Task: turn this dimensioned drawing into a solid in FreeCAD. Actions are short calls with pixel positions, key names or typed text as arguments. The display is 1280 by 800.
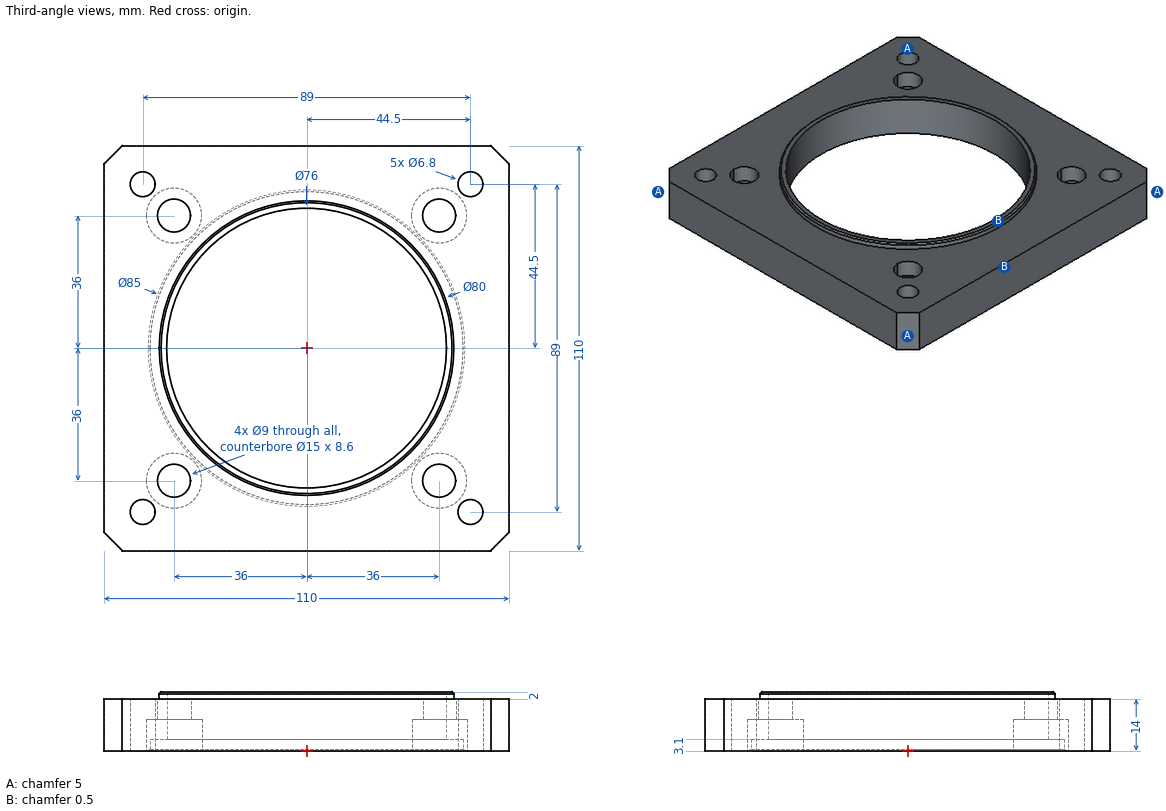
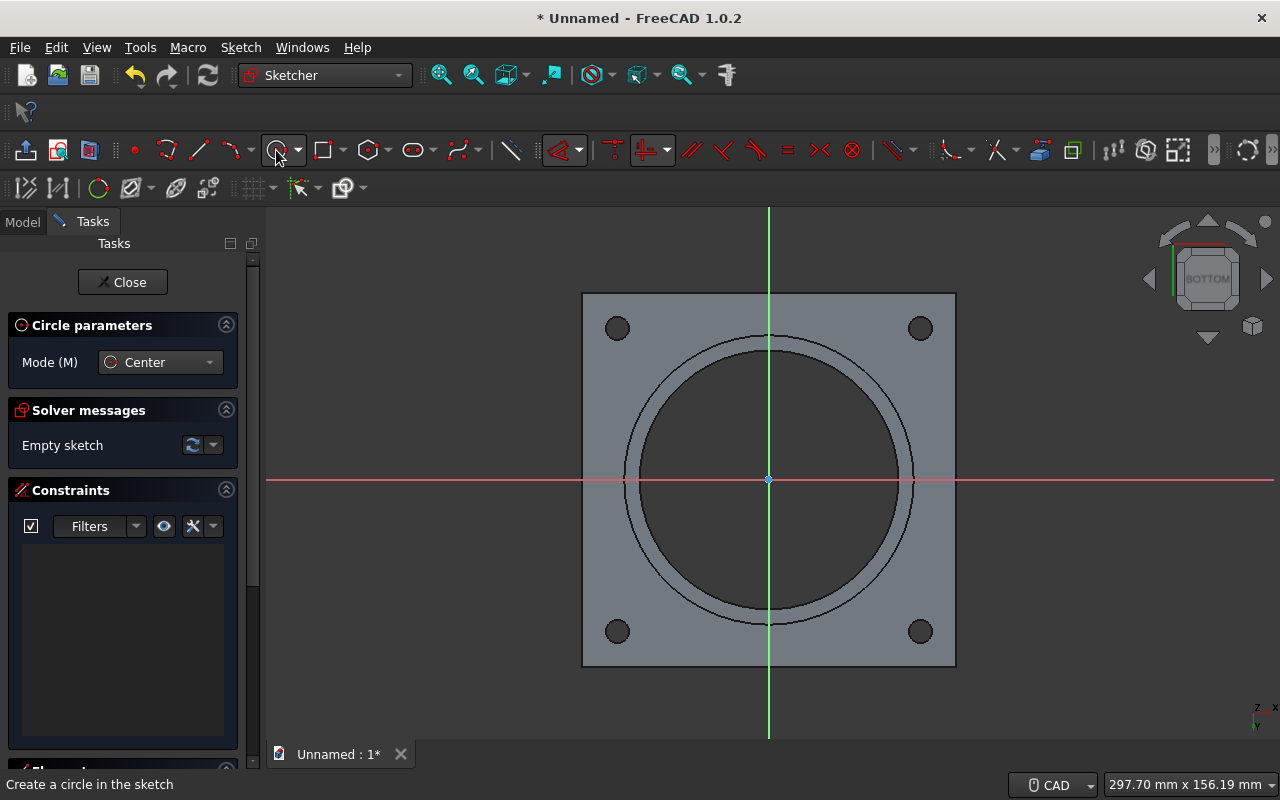
scroll(646, 357, up, 2)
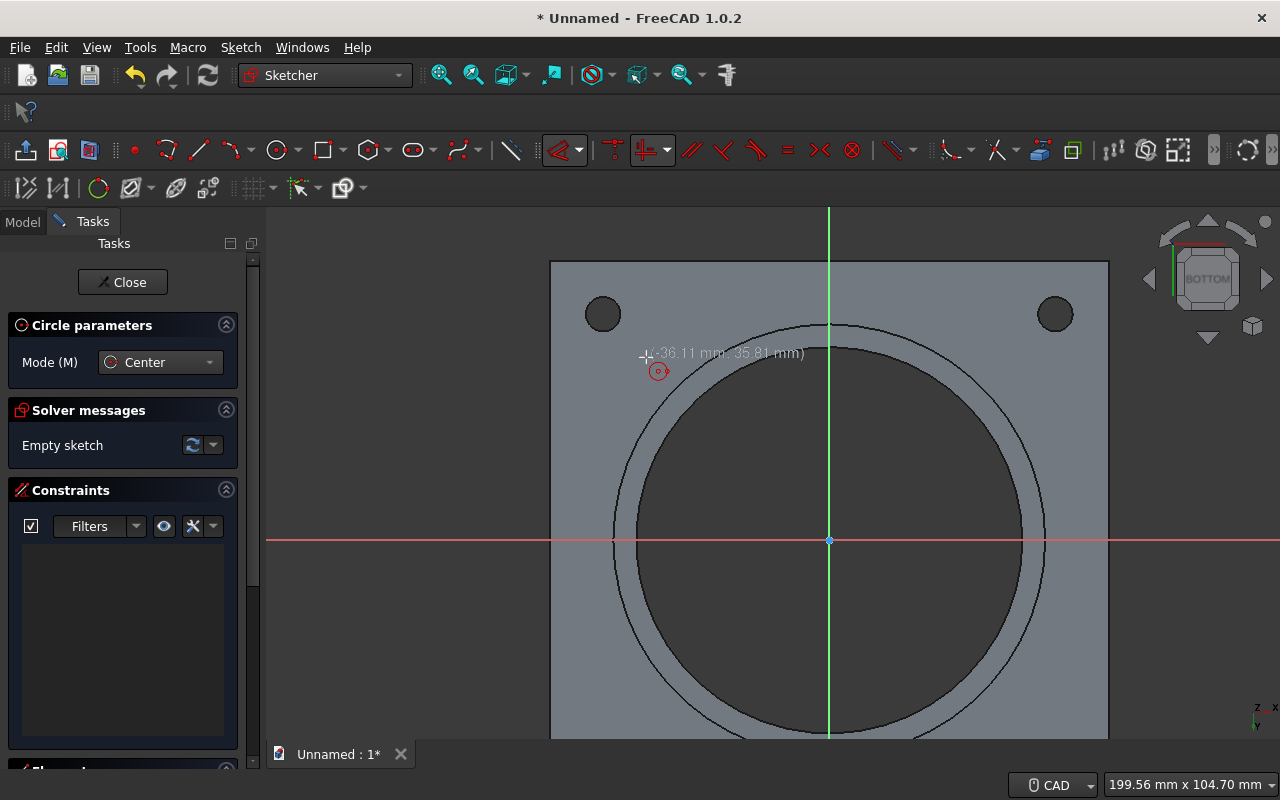
click(646, 357)
click(663, 341)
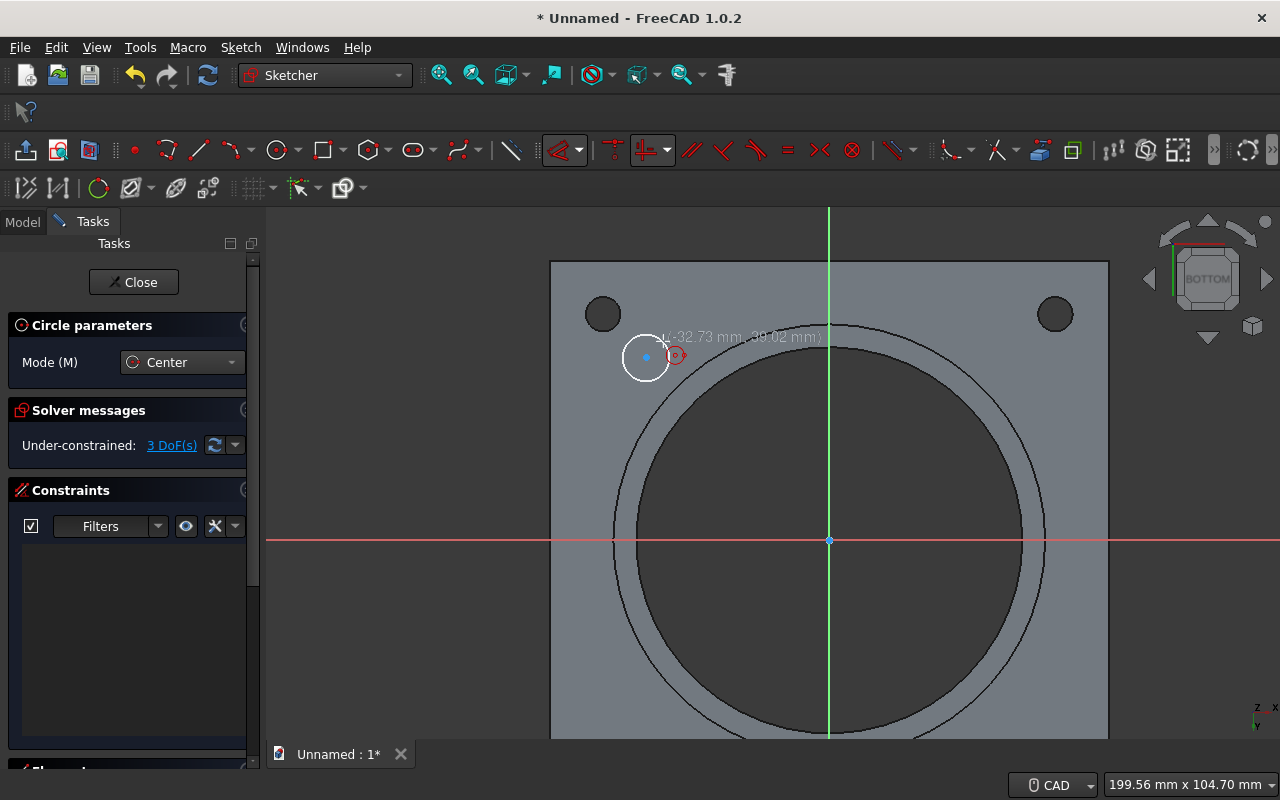
scroll(294, 235, down, 1)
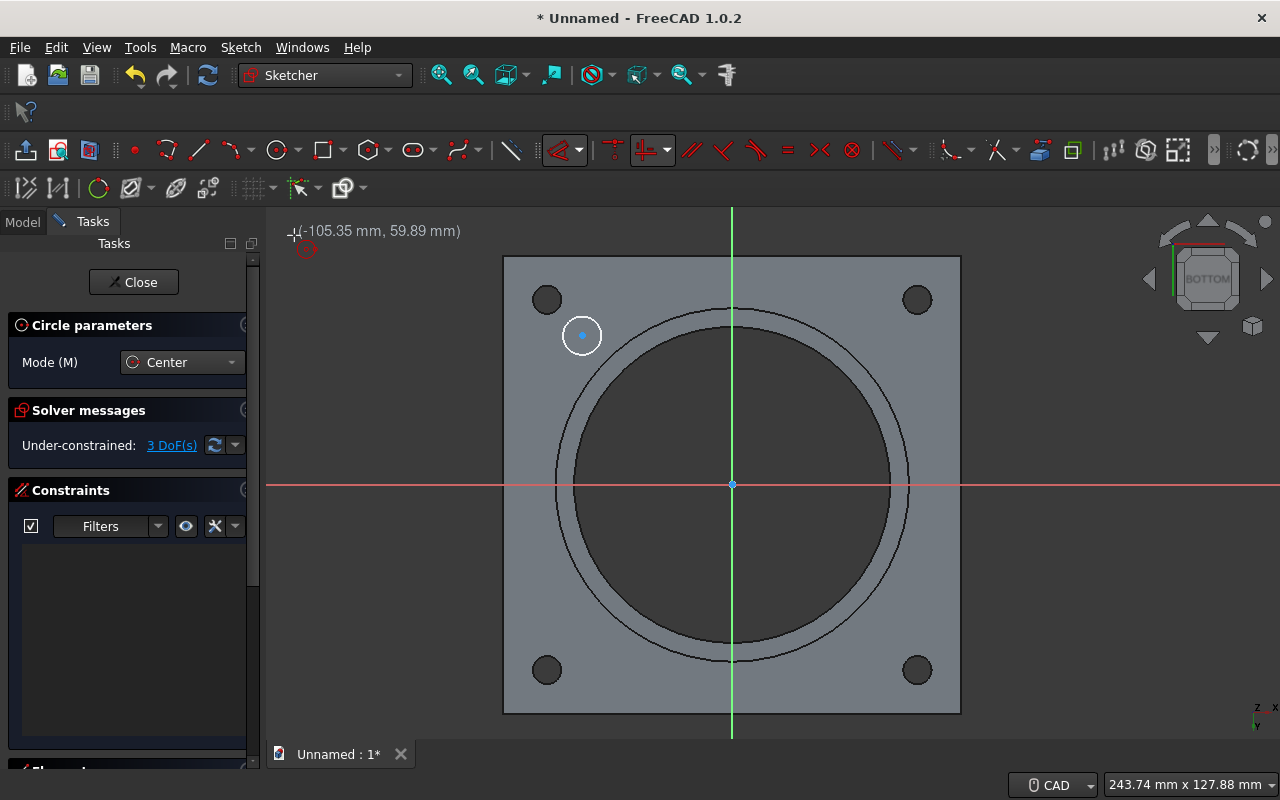
click(582, 635)
click(596, 621)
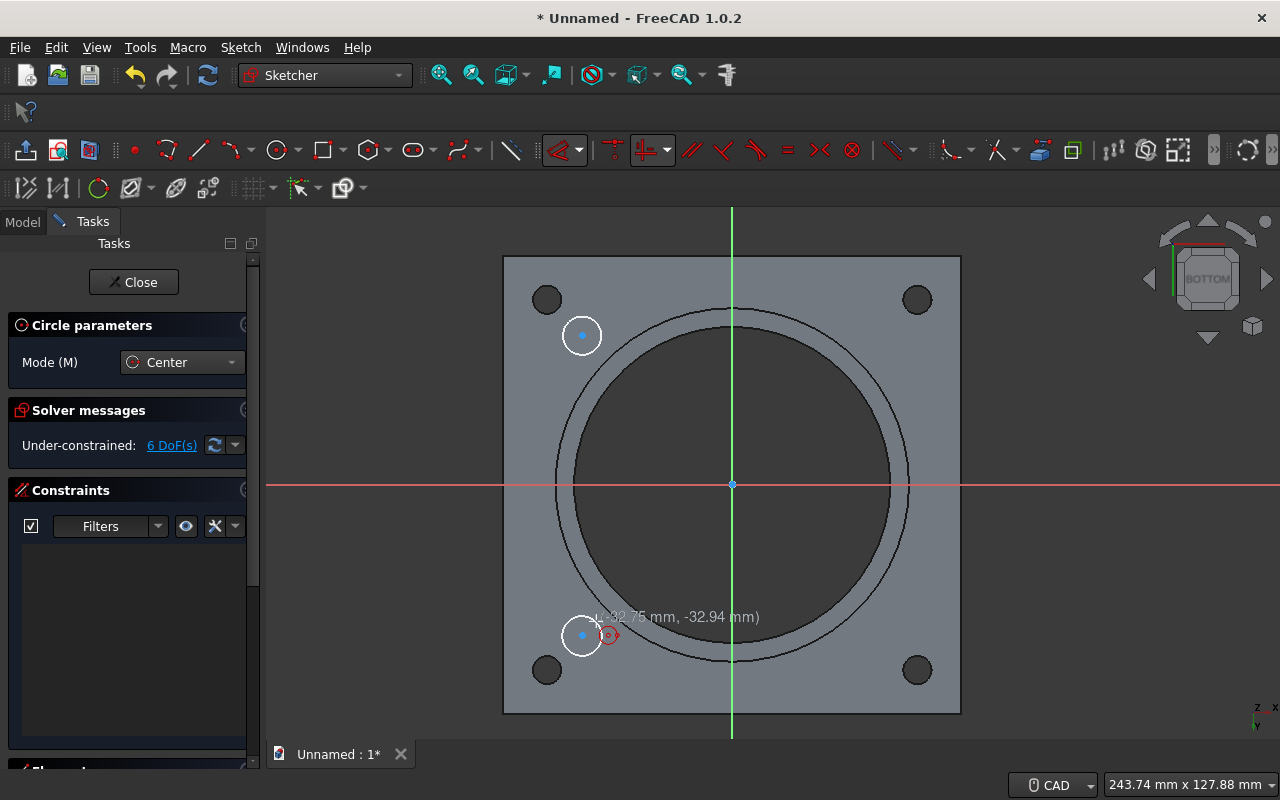
click(882, 335)
click(895, 322)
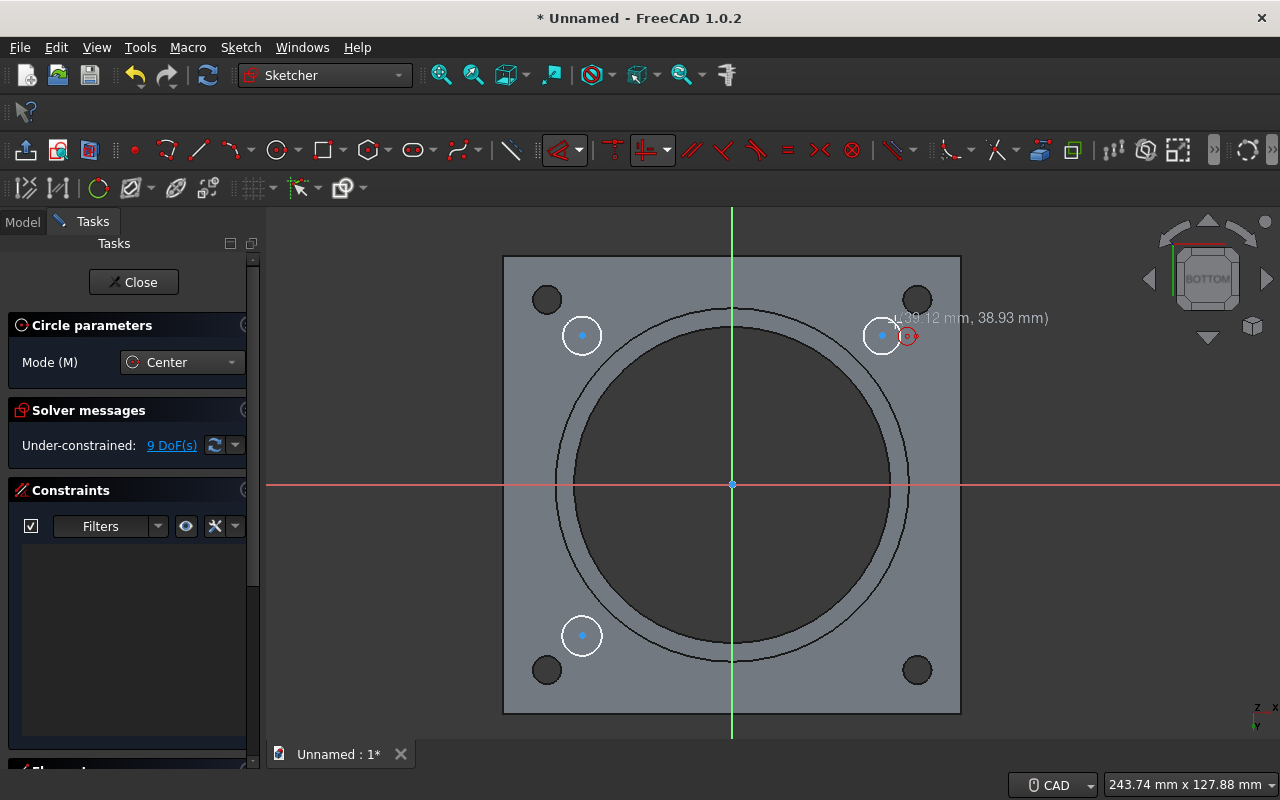
click(882, 635)
click(895, 621)
key(Escape)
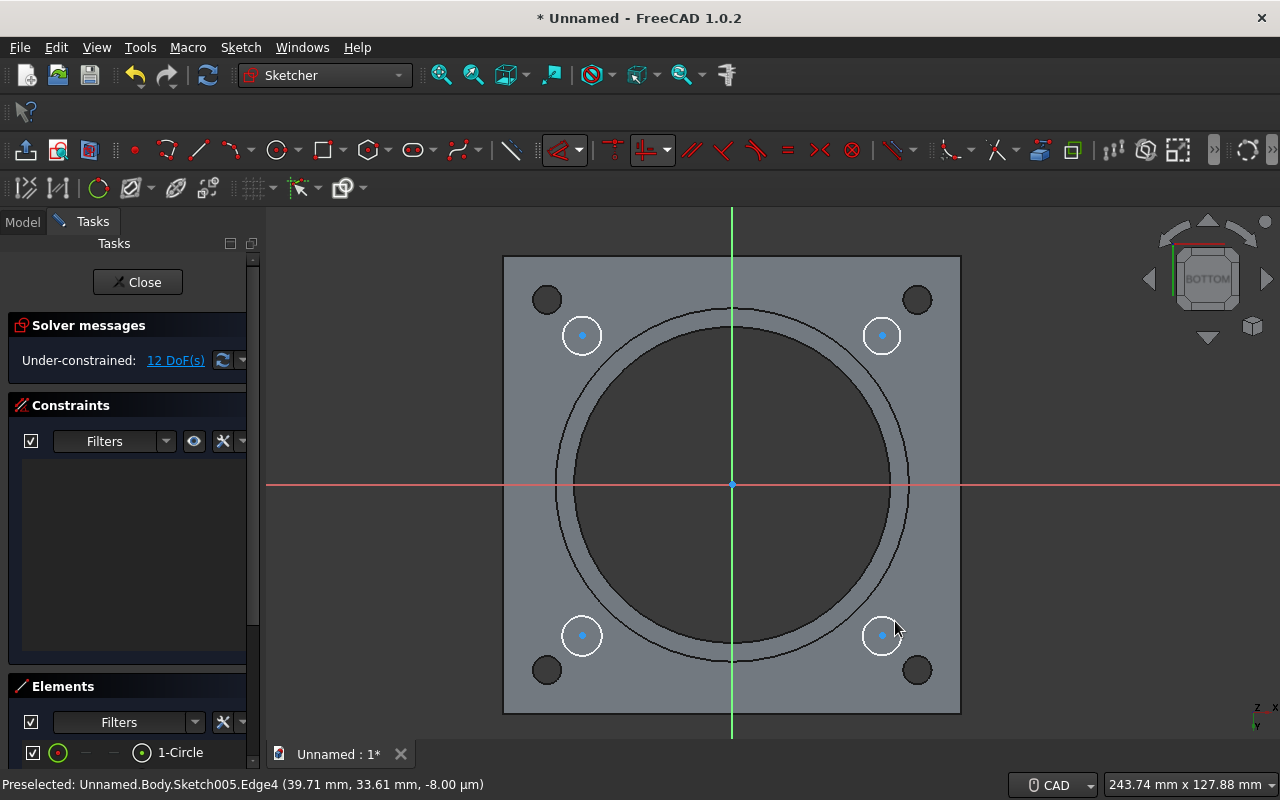
click(596, 322)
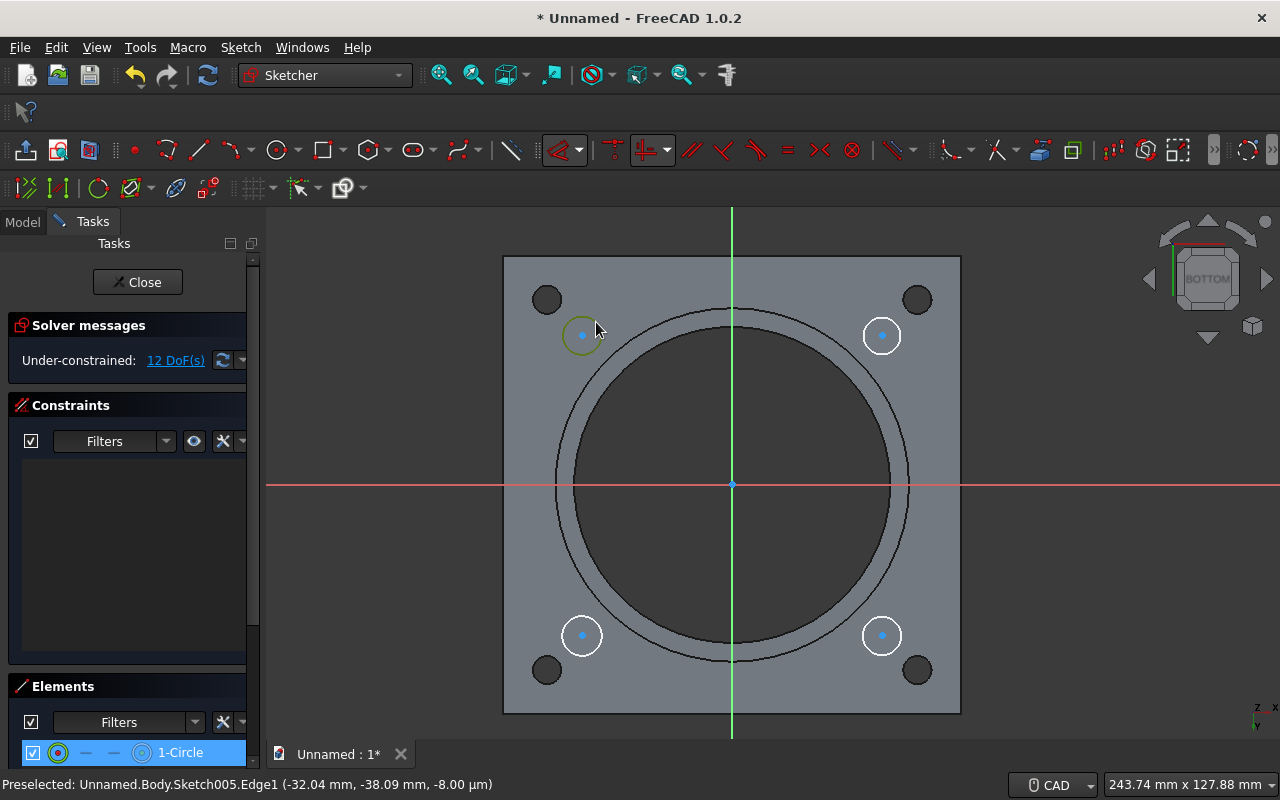
click(596, 622)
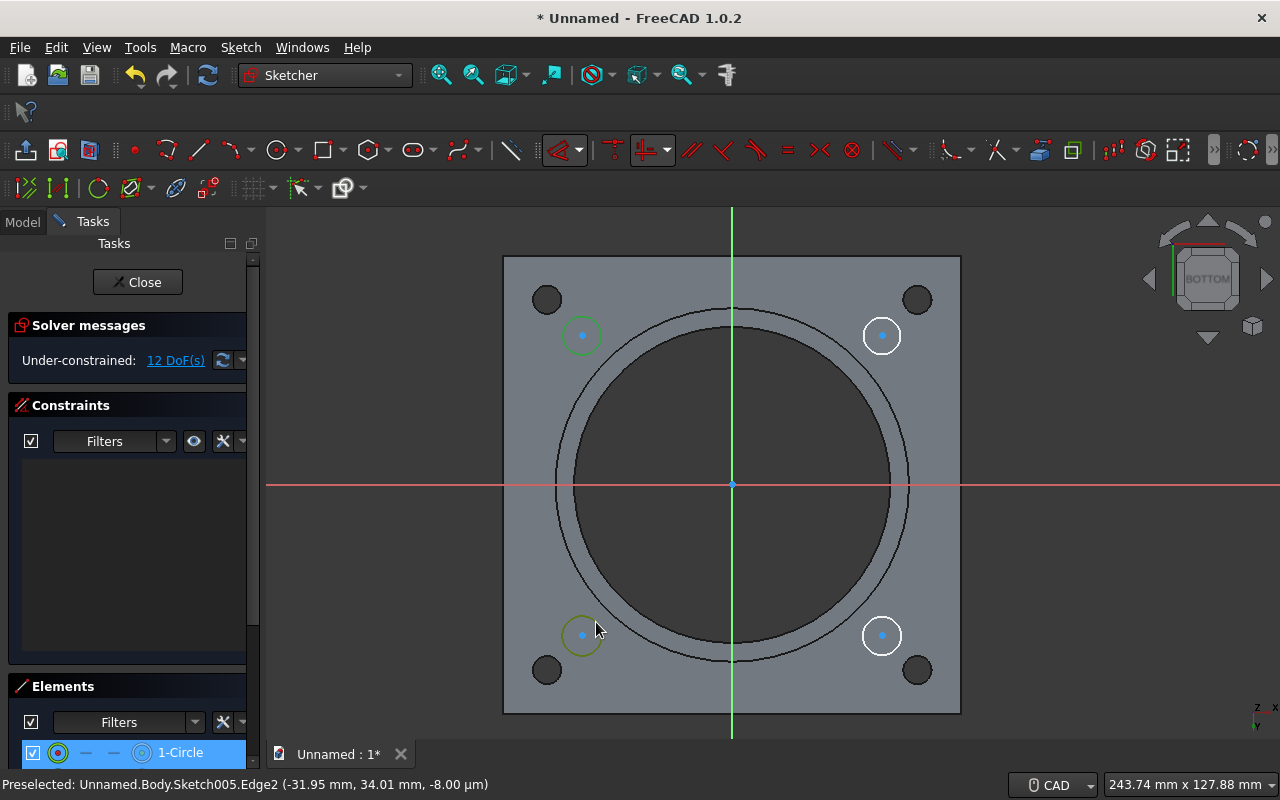
click(895, 323)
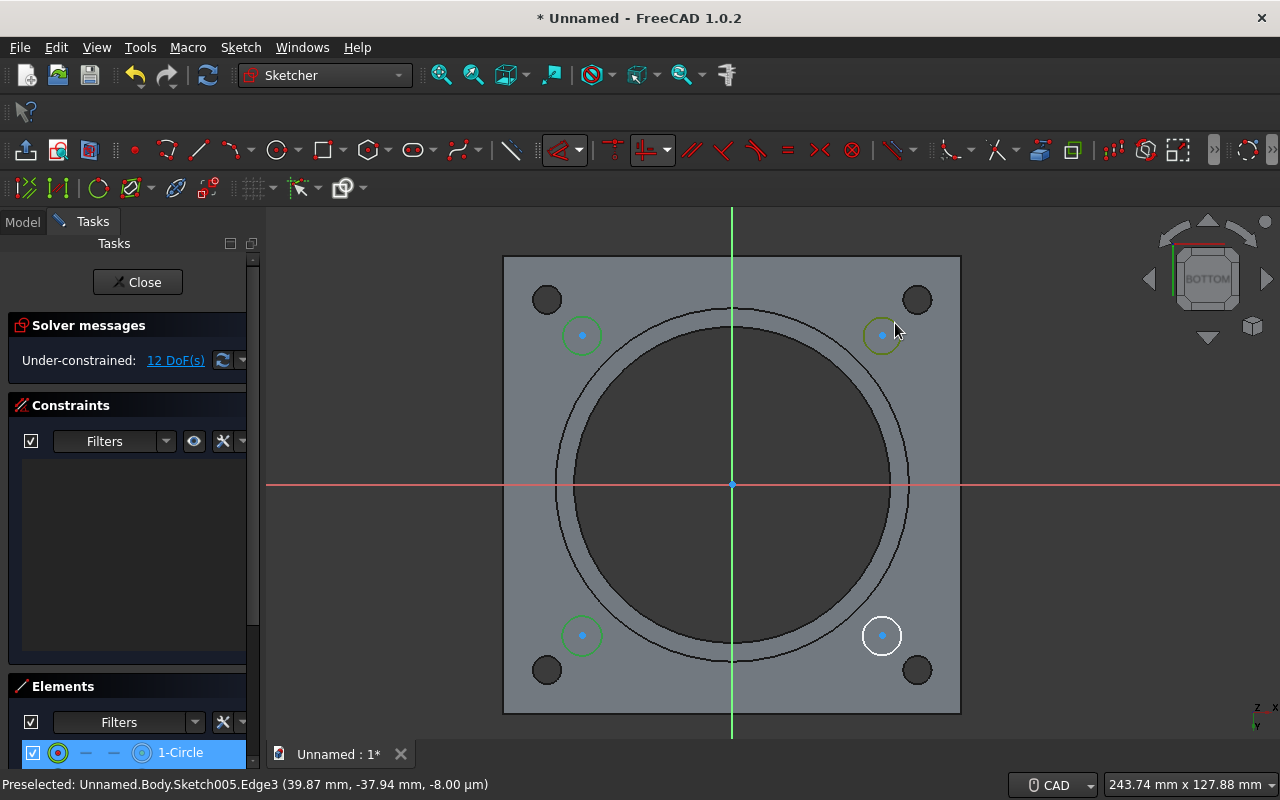
click(895, 622)